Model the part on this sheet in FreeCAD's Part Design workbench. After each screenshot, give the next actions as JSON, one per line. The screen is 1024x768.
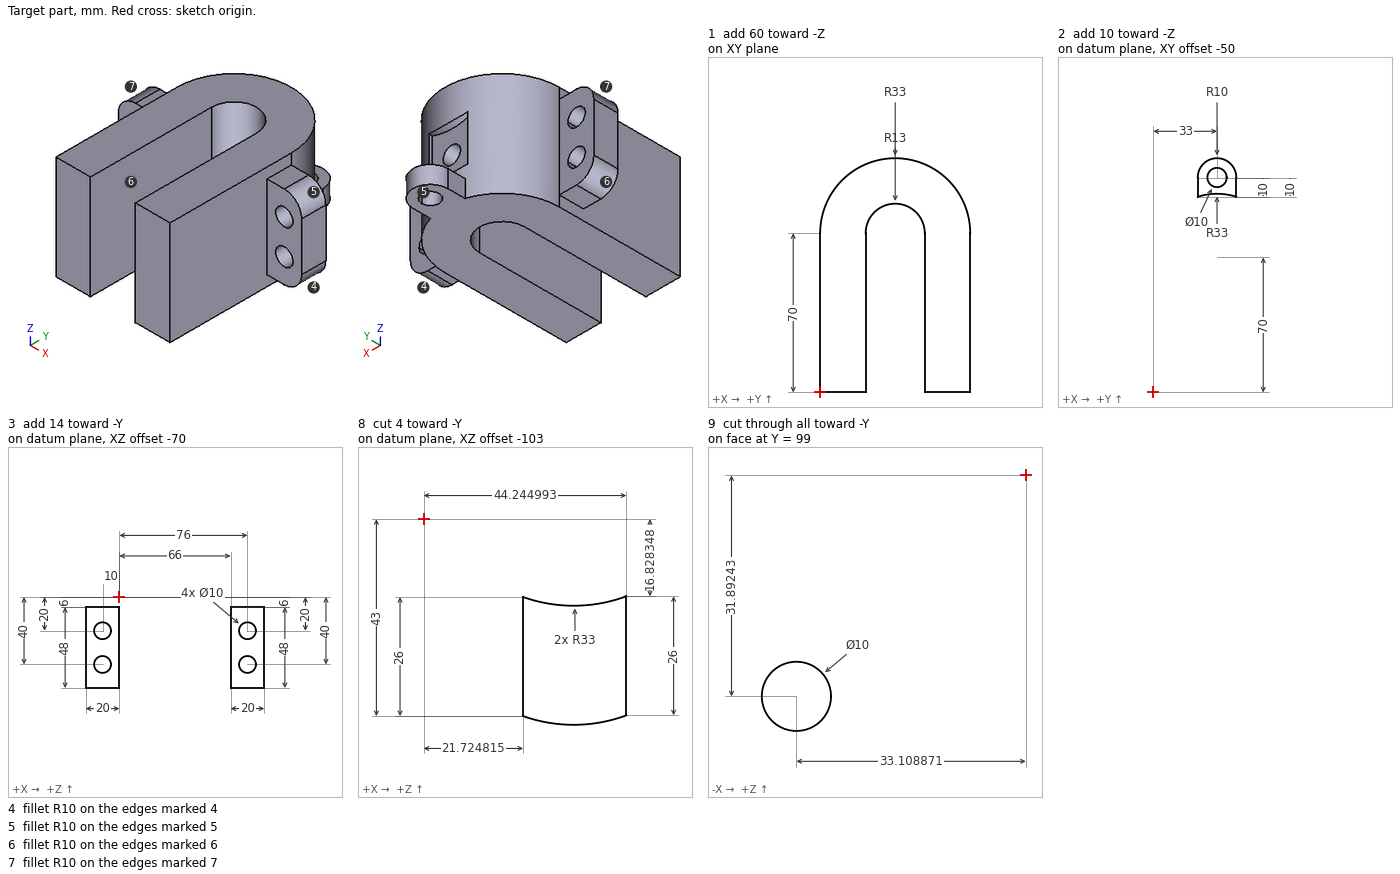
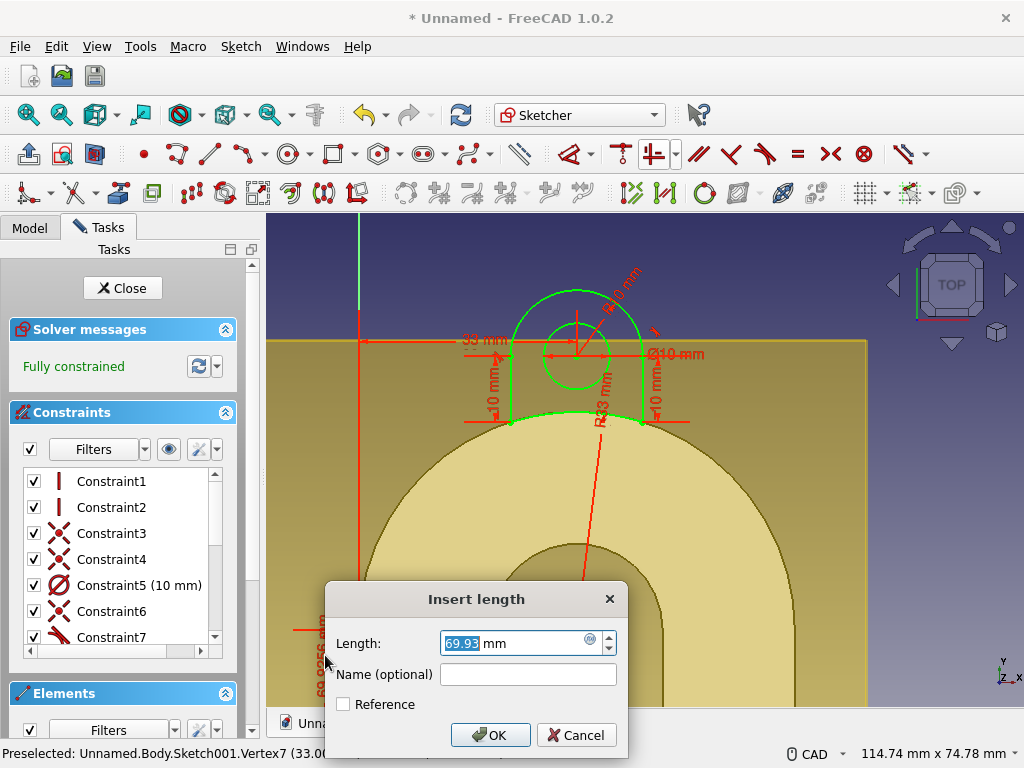
{"action": "type", "text": "70"}
{"action": "key", "text": "Return"}
{"action": "key", "text": "Escape"}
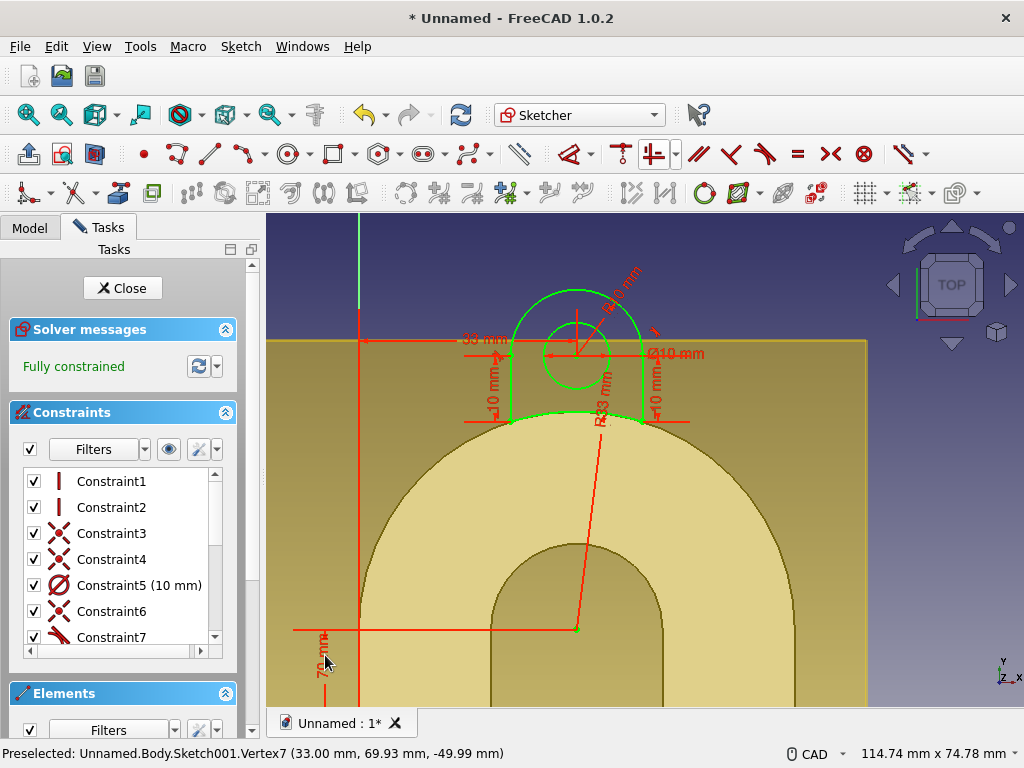
{"action": "left_click", "coordinate": [123, 288]}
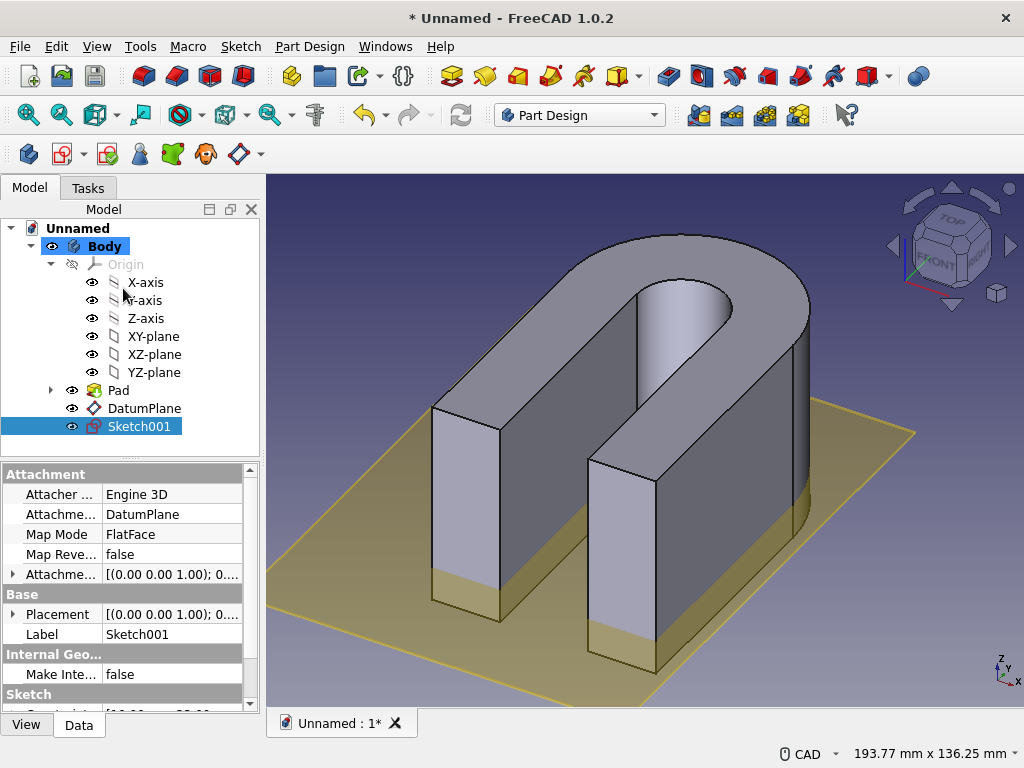
{"action": "left_click", "coordinate": [452, 76]}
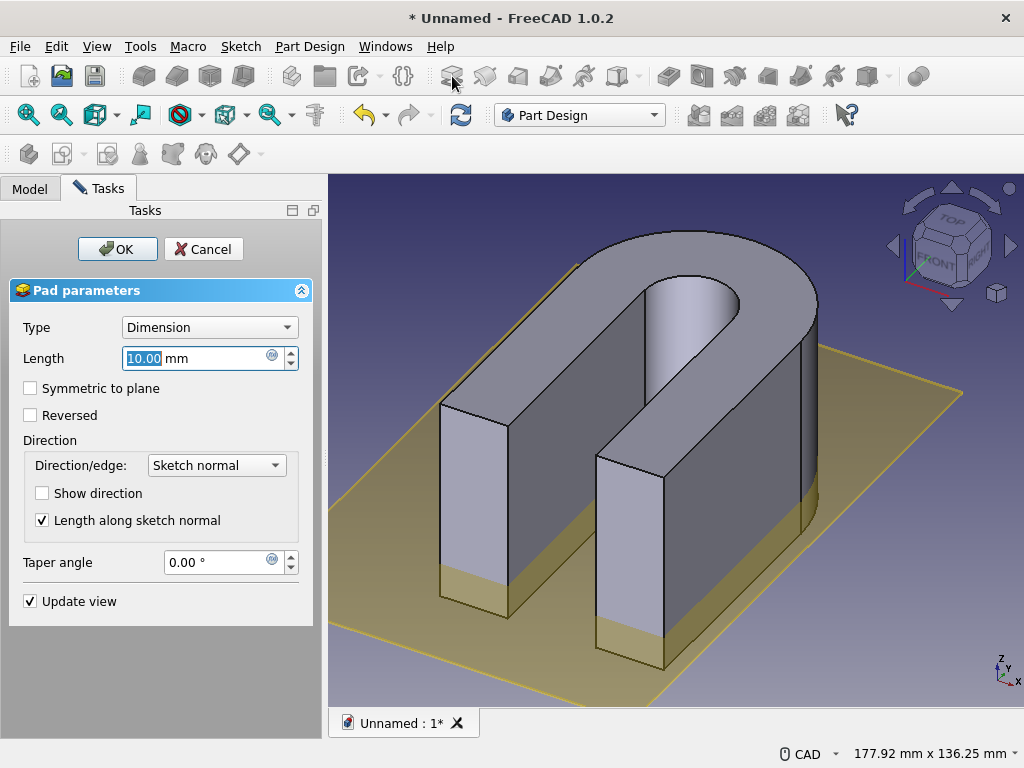
{"action": "type", "text": "10"}
{"action": "key", "text": "Tab"}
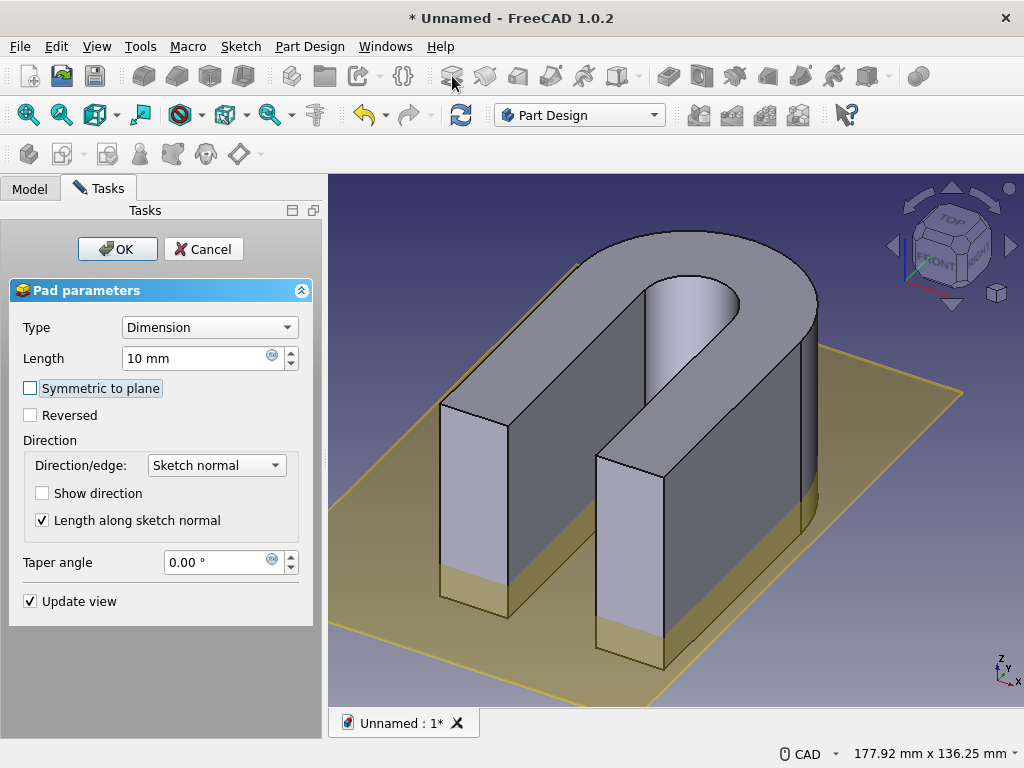
{"action": "left_click", "coordinate": [31, 415]}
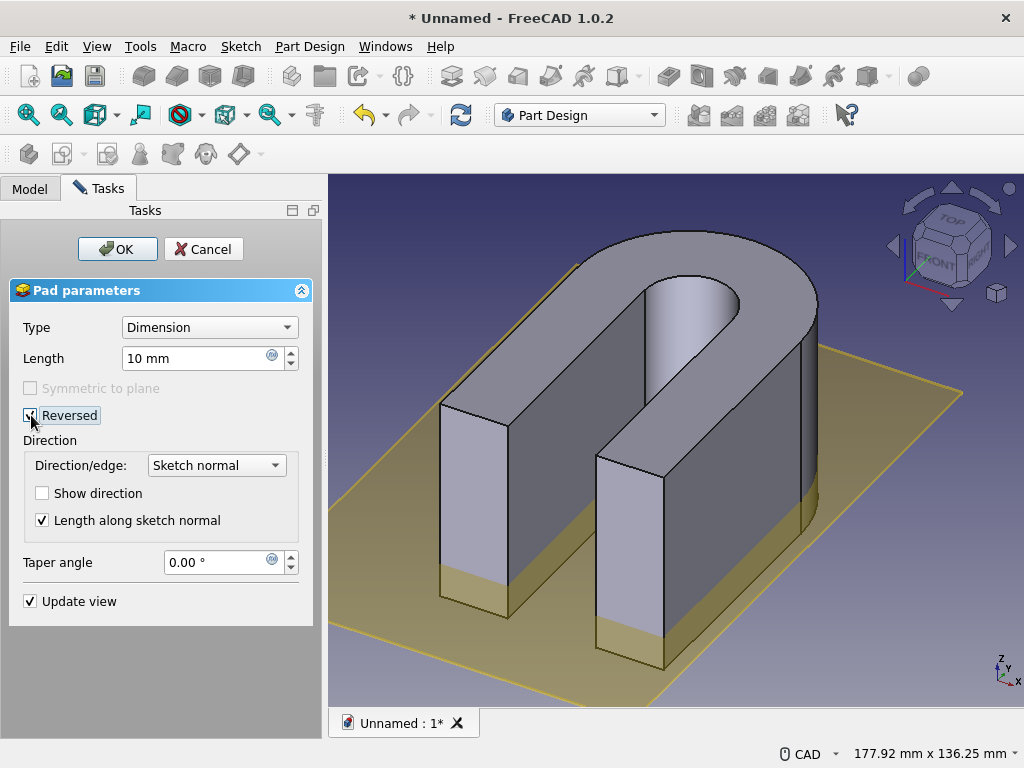
{"action": "left_click", "coordinate": [118, 249]}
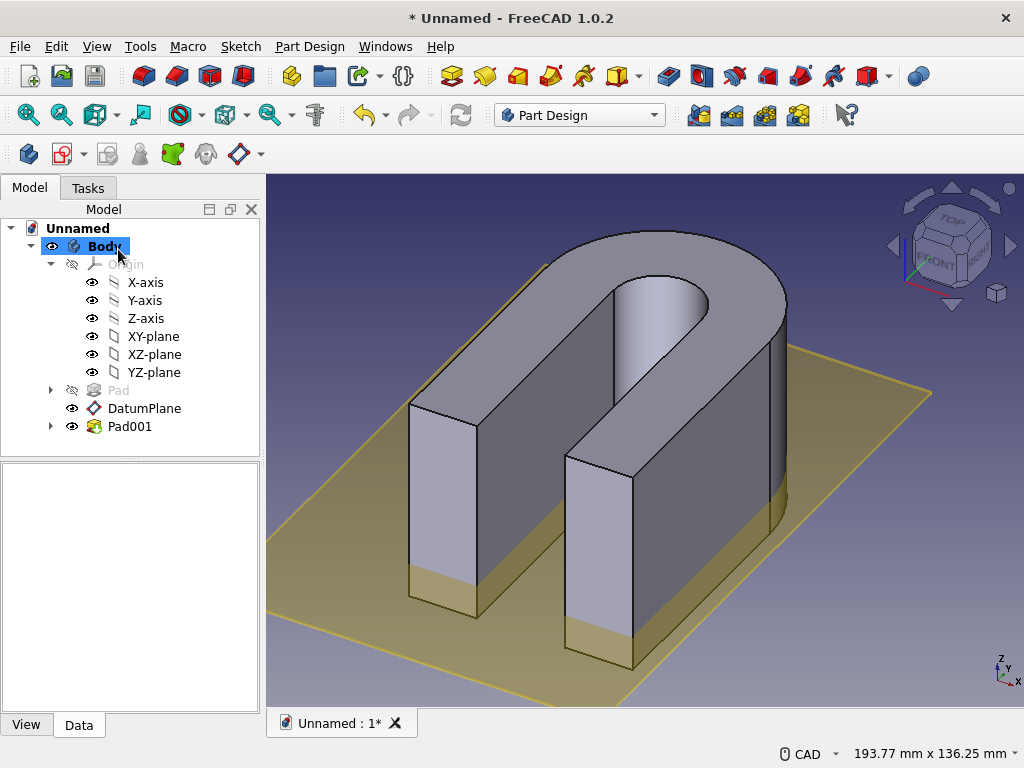
{"action": "left_click", "coordinate": [117, 408]}
{"action": "key", "text": "space"}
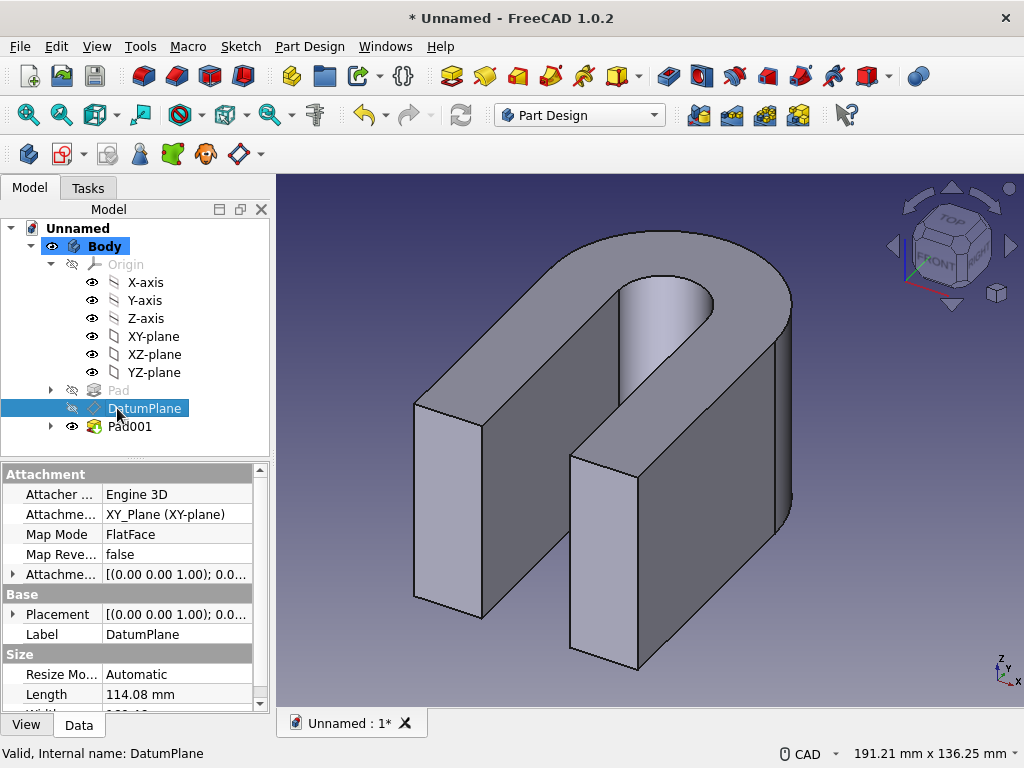
{"action": "left_click", "coordinate": [29, 116]}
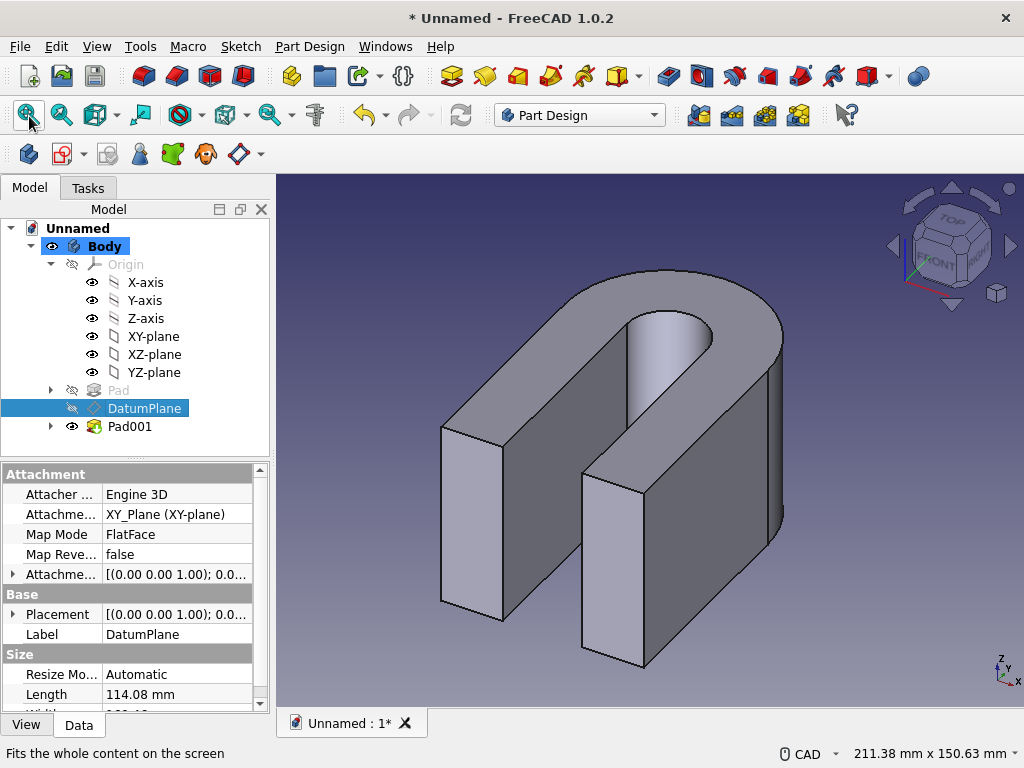
{"action": "left_click", "coordinate": [137, 354]}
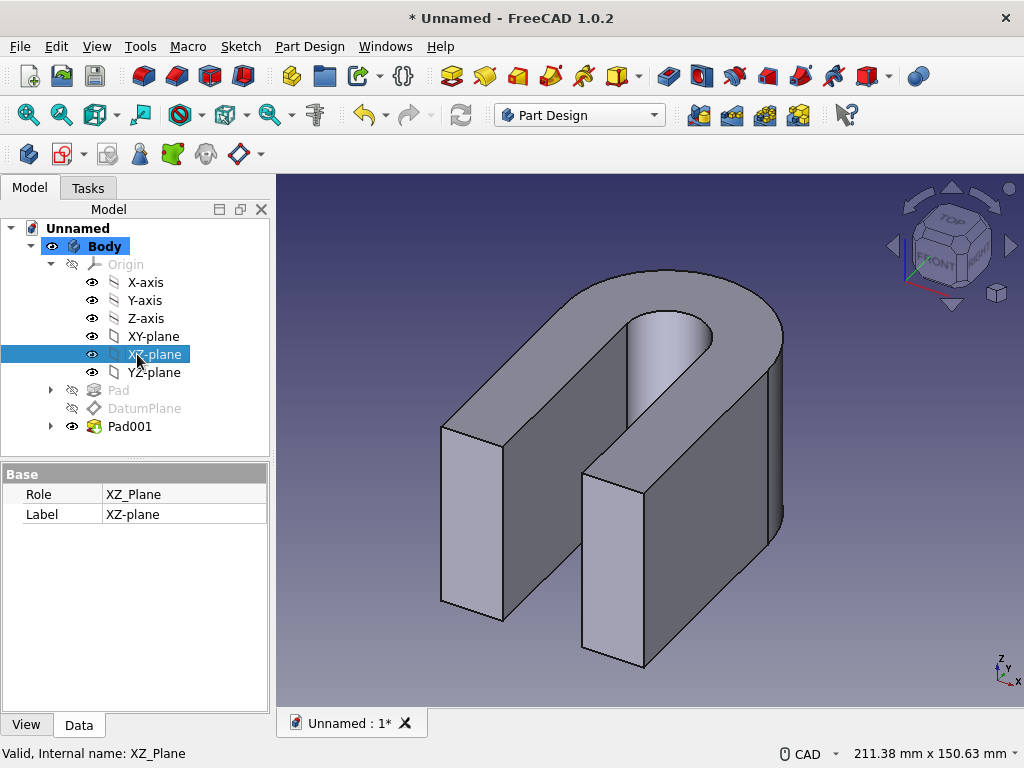
{"action": "left_click", "coordinate": [238, 154]}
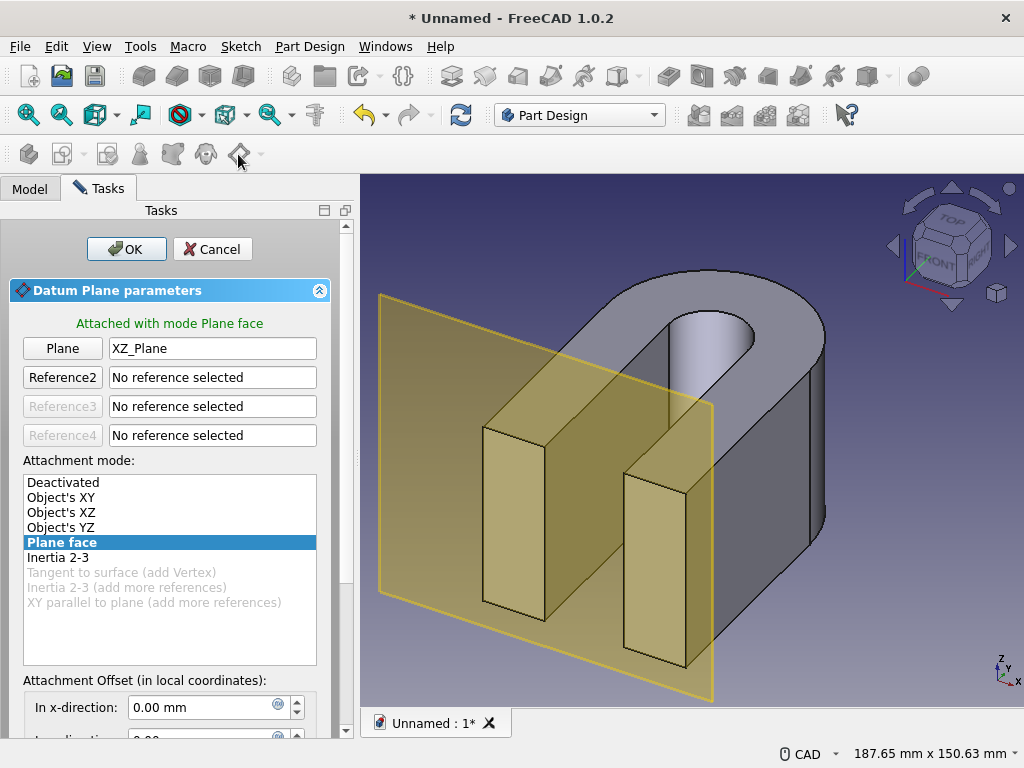
{"action": "scroll", "coordinate": [346, 479], "scroll_direction": "down", "scroll_amount": 2}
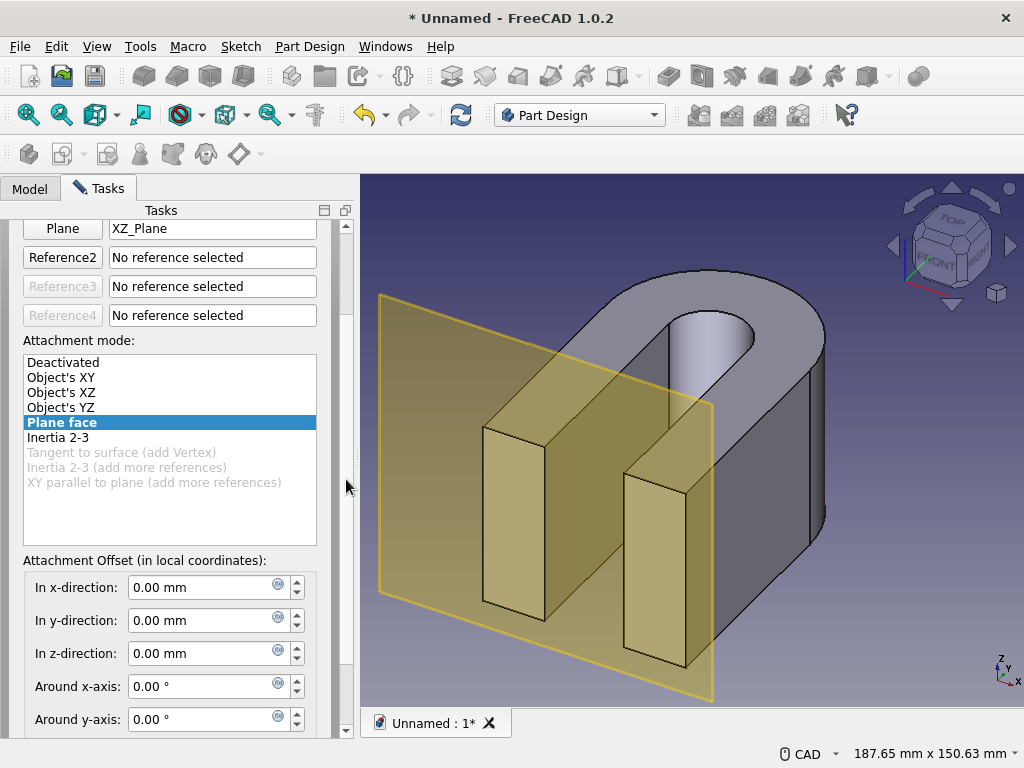
{"action": "triple_click", "coordinate": [210, 654]}